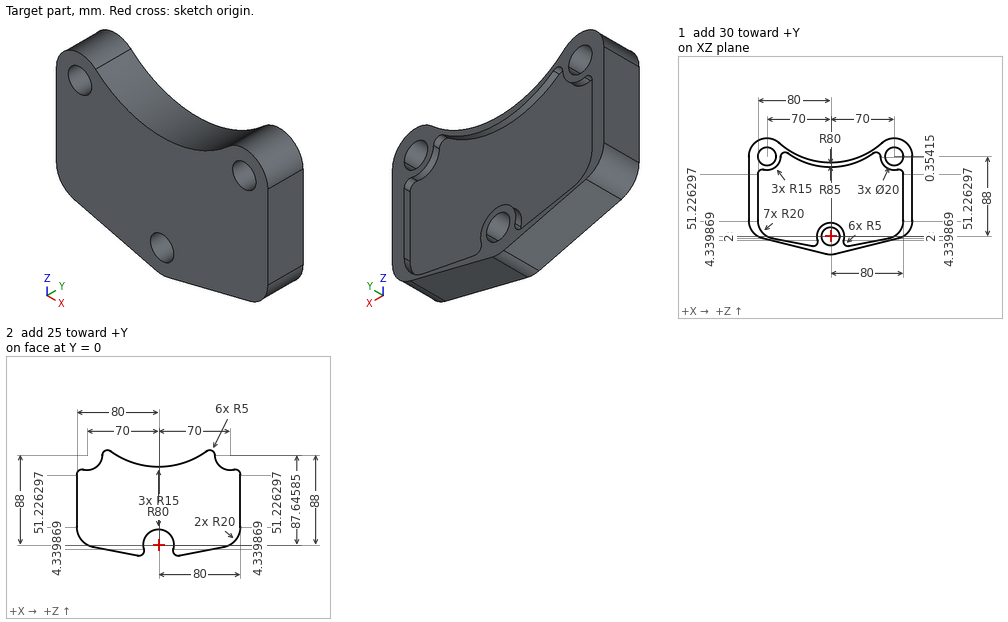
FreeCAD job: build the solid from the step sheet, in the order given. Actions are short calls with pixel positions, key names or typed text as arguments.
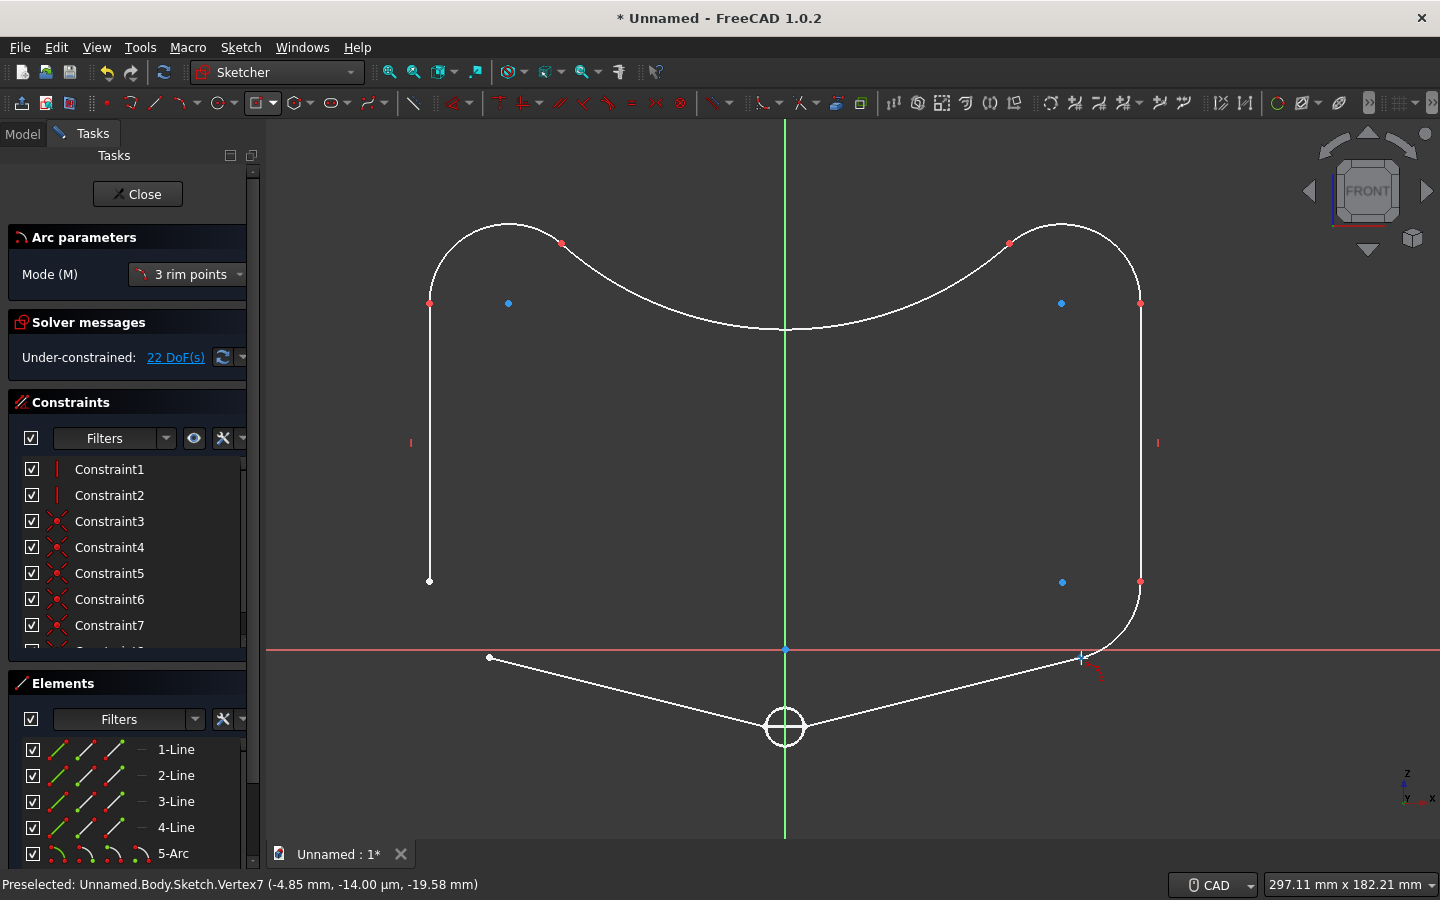
scroll(781, 729, up, 10)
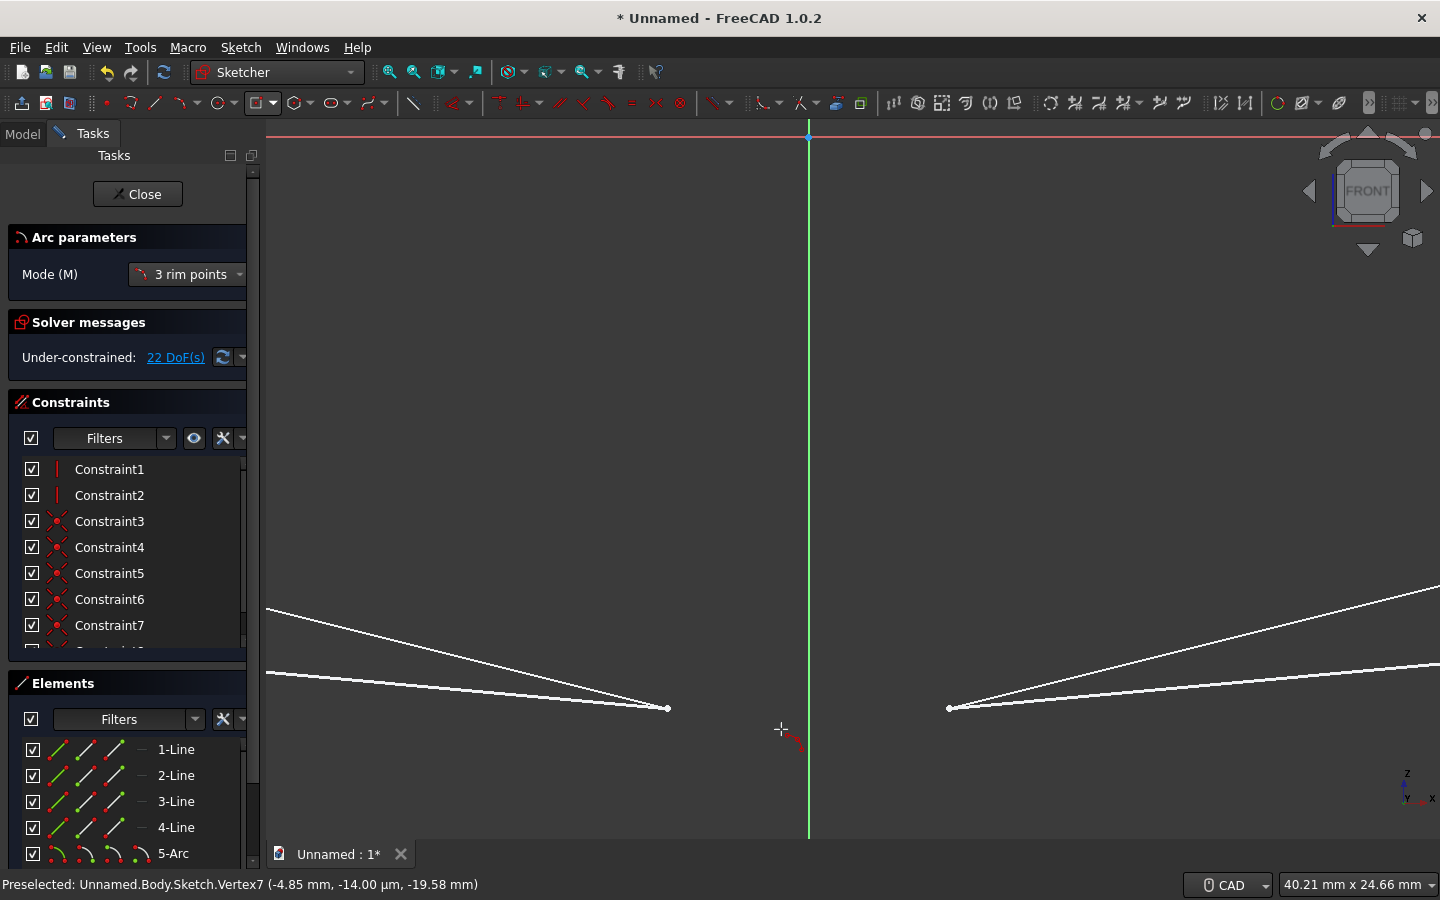
click(780, 720)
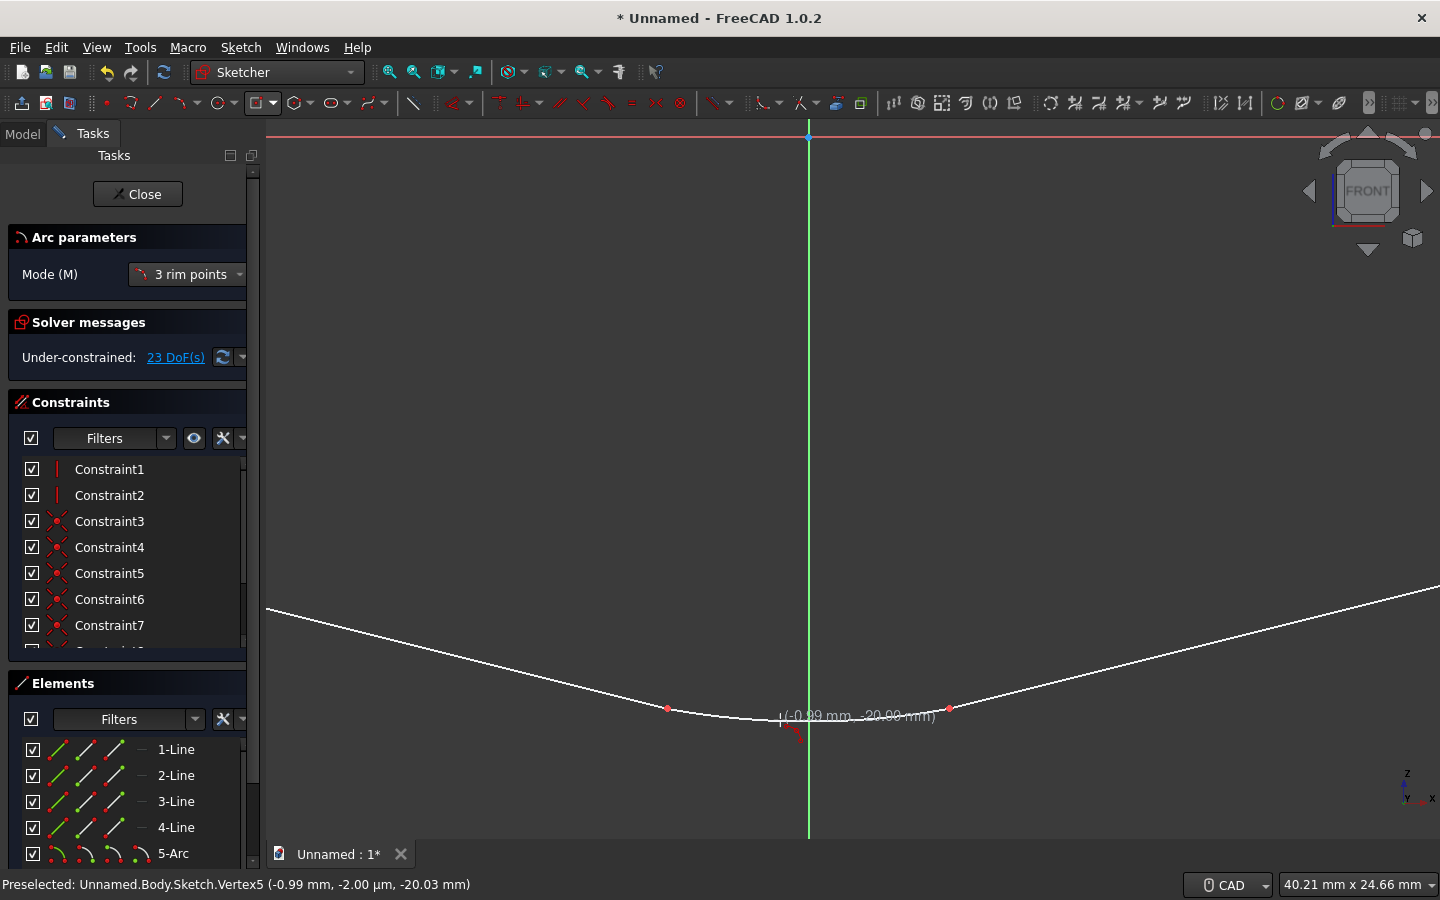
scroll(781, 730, down, 10)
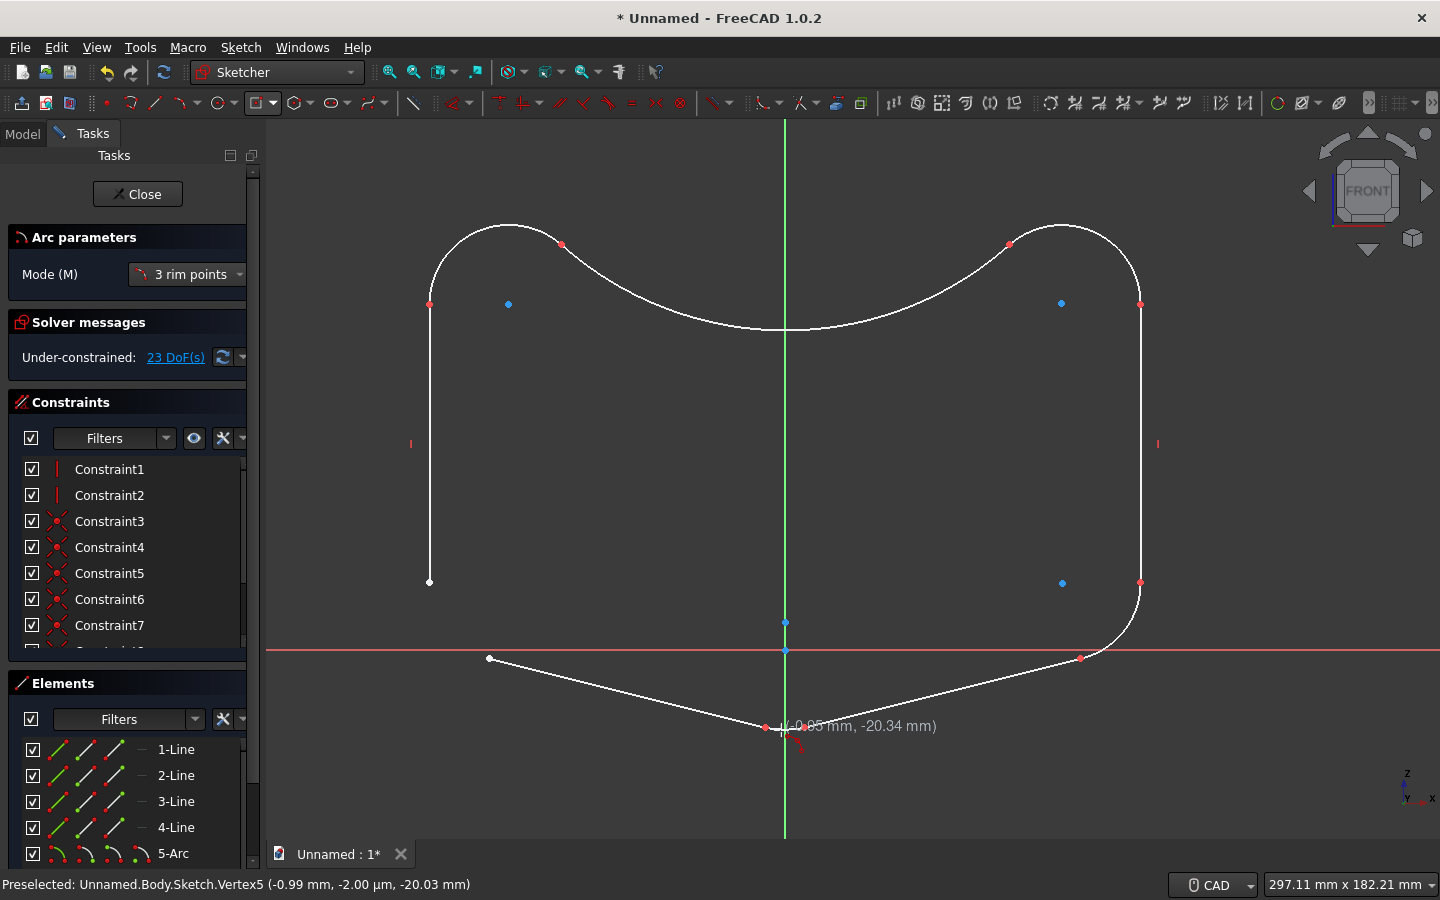
scroll(489, 658, up, 4)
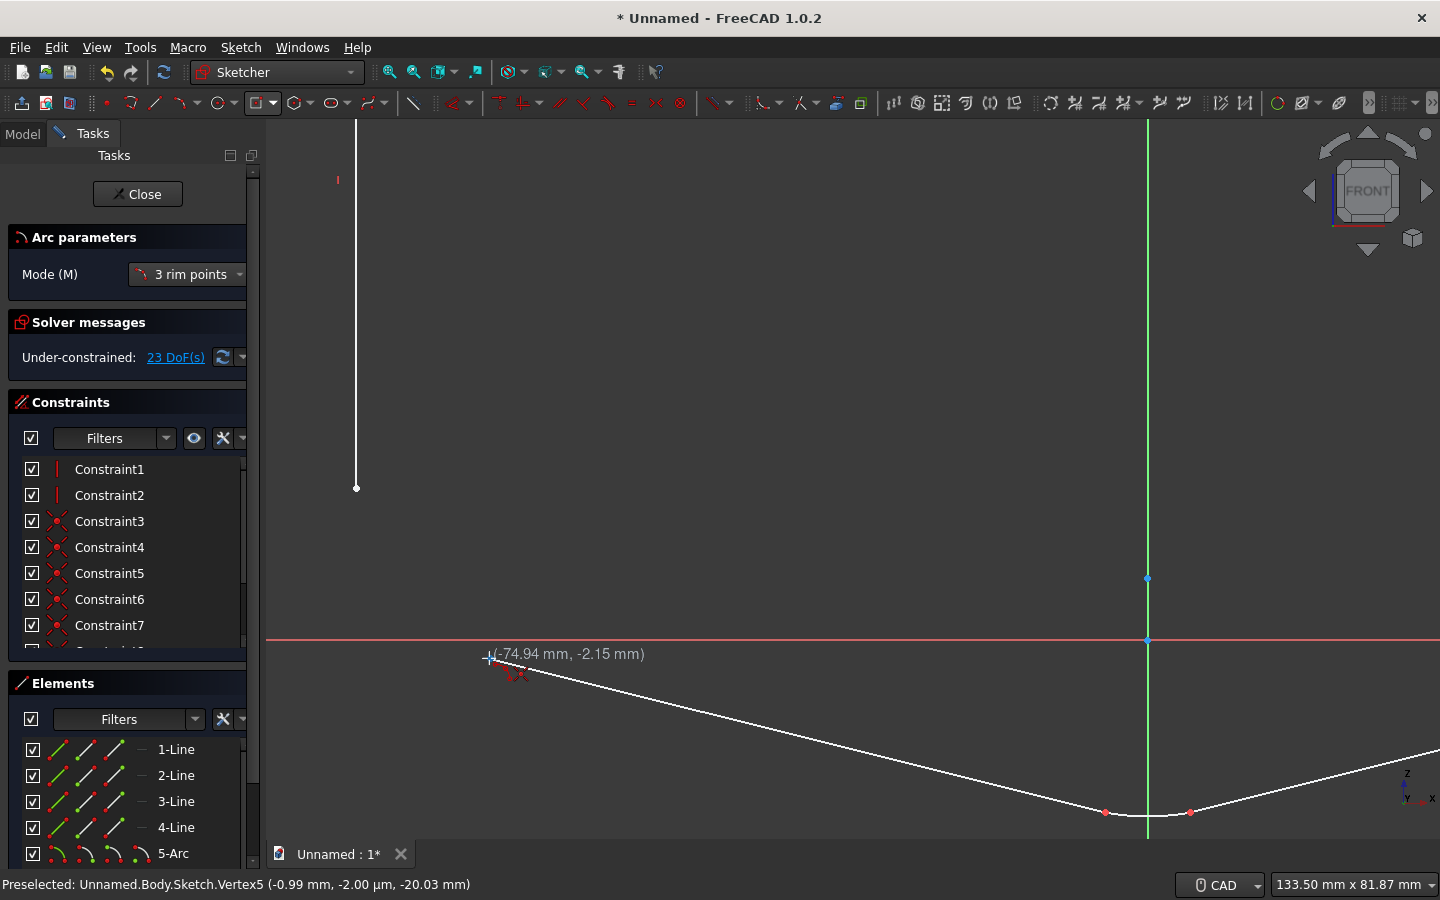
click(490, 659)
click(356, 489)
click(394, 596)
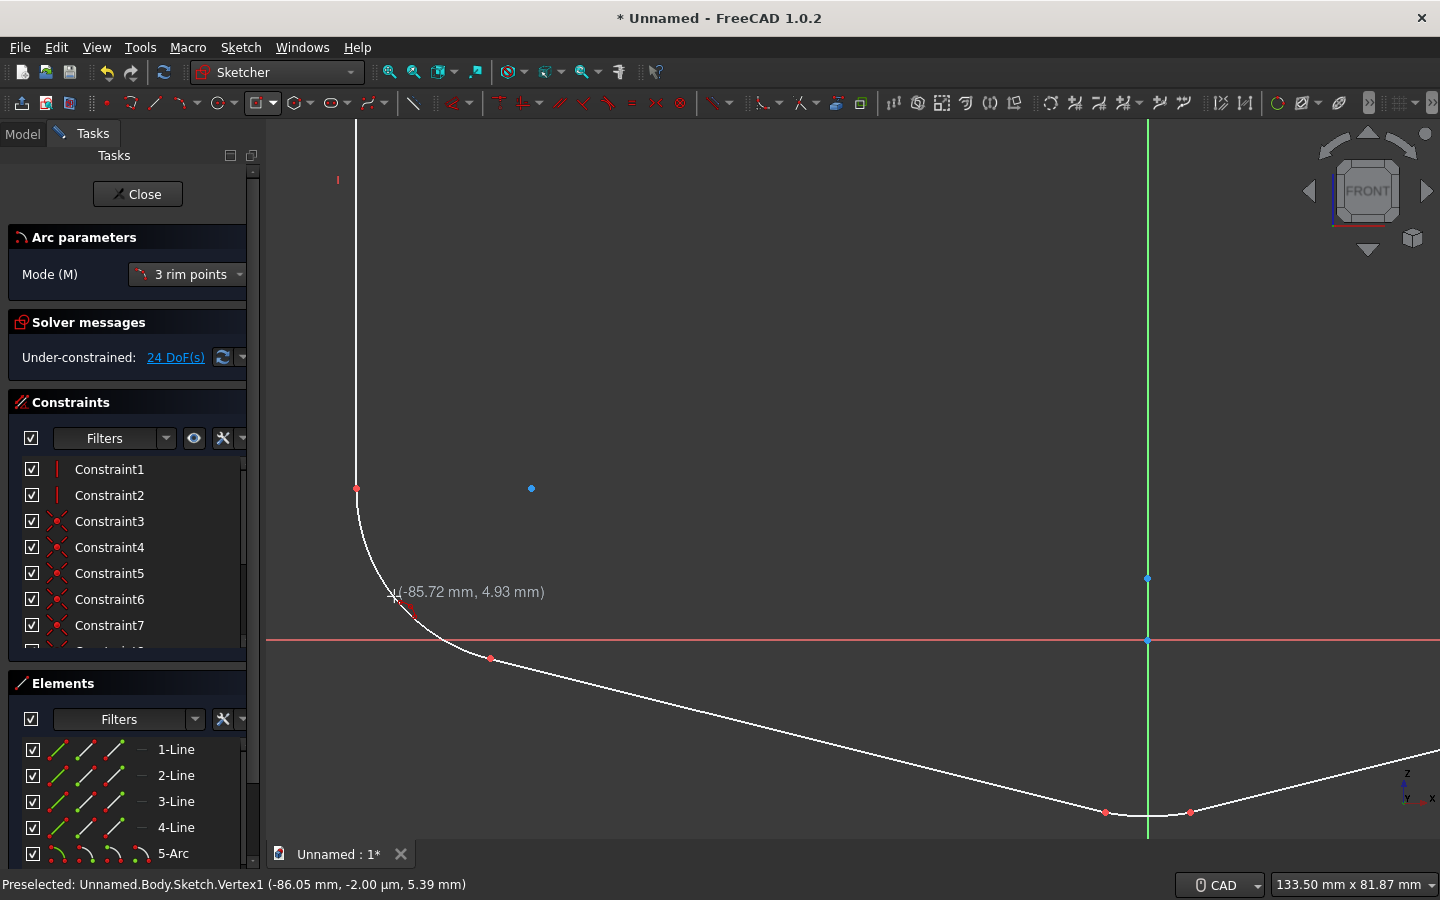
click(156, 104)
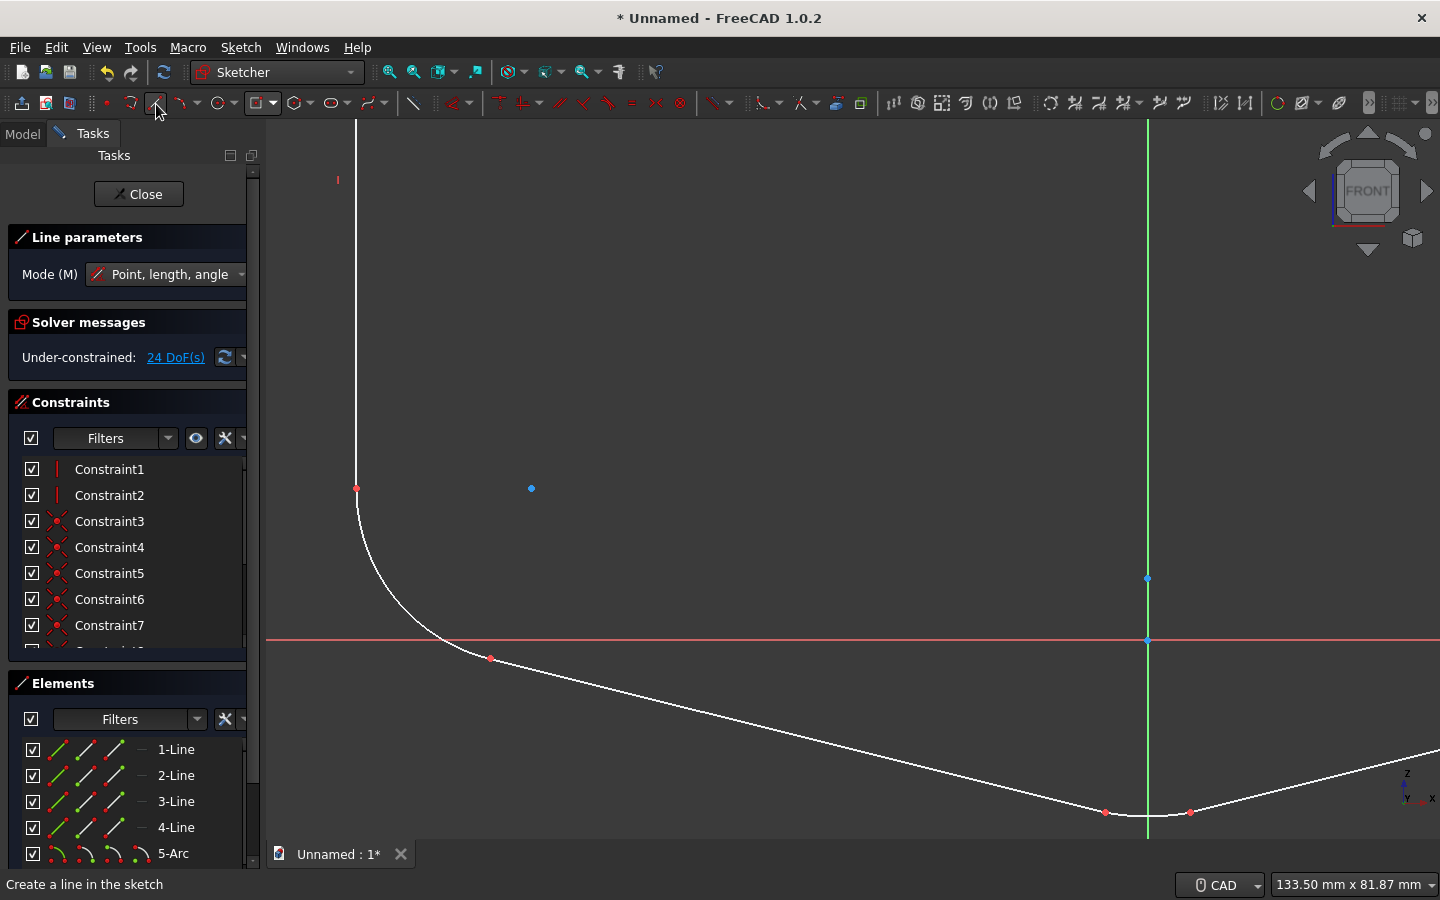
scroll(488, 657, down, 4)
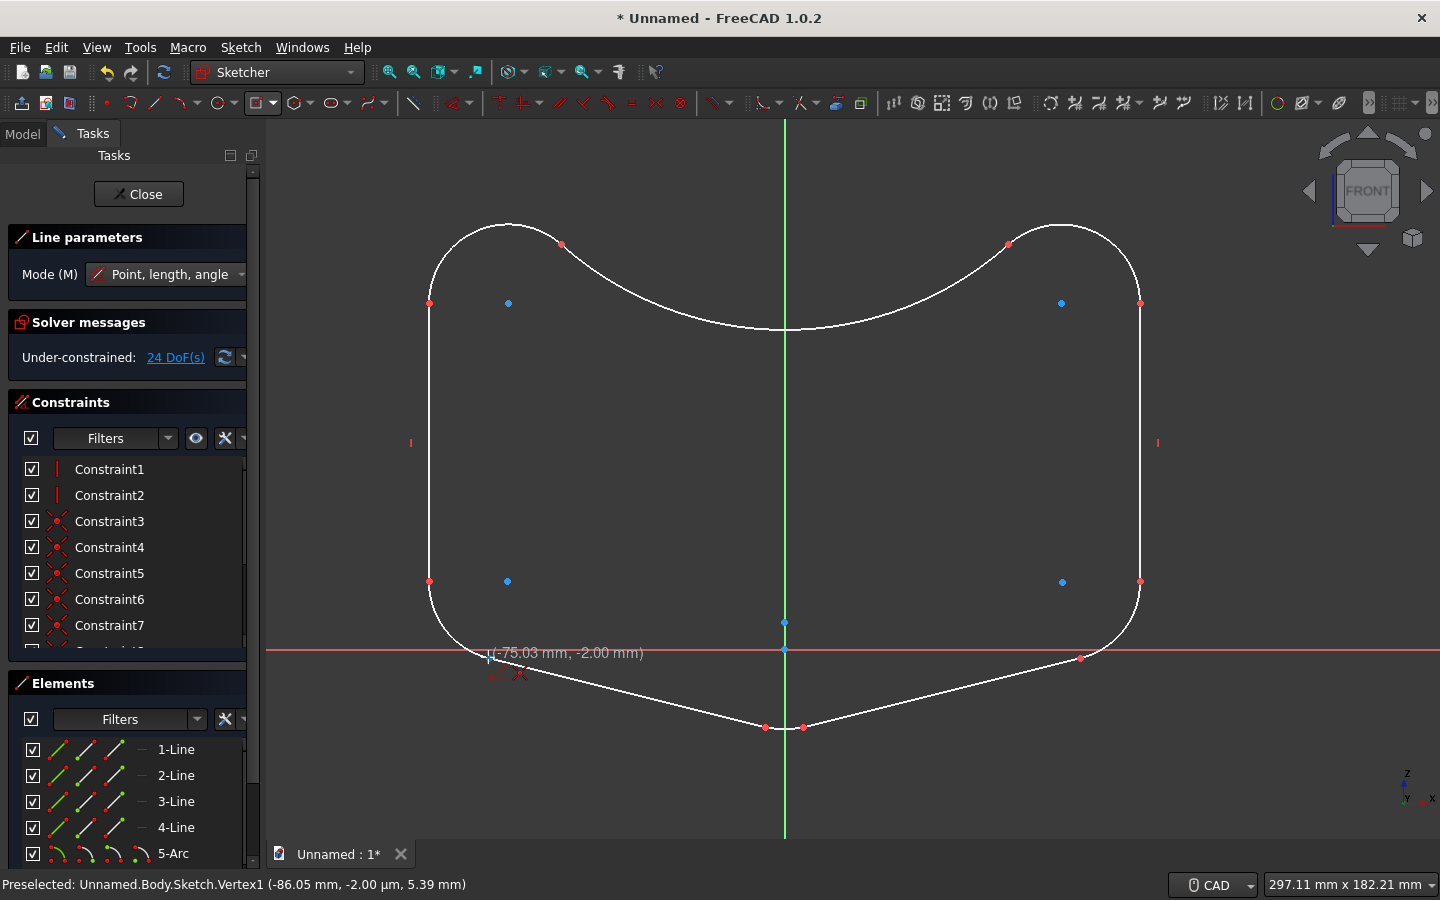
click(468, 379)
click(468, 581)